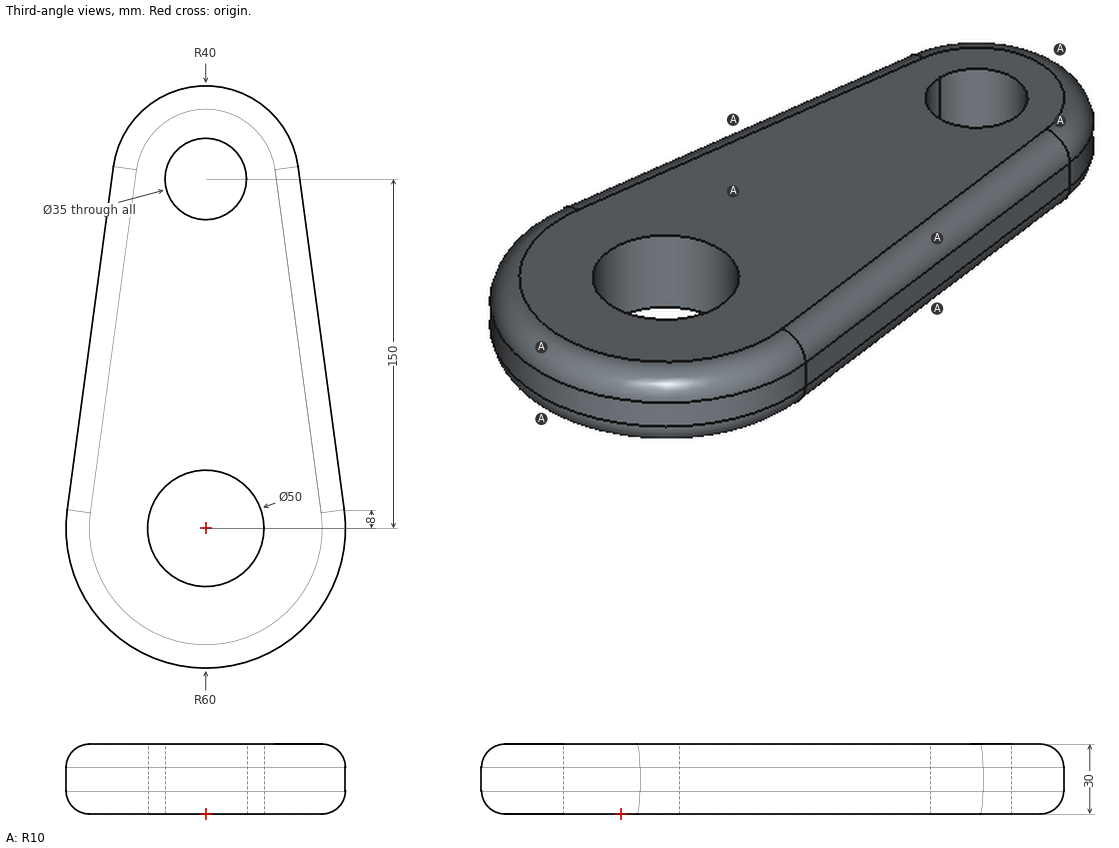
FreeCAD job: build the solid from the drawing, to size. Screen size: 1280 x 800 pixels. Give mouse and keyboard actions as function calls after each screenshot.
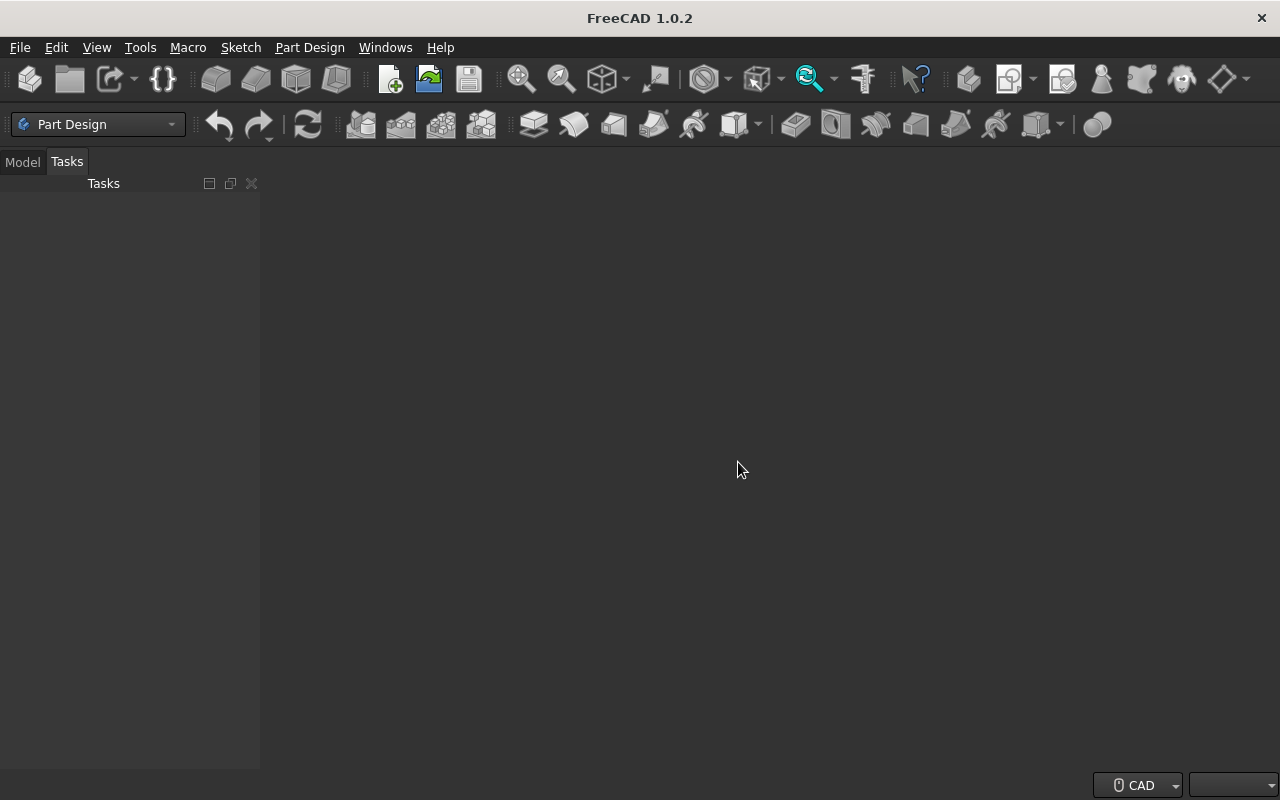
click(390, 80)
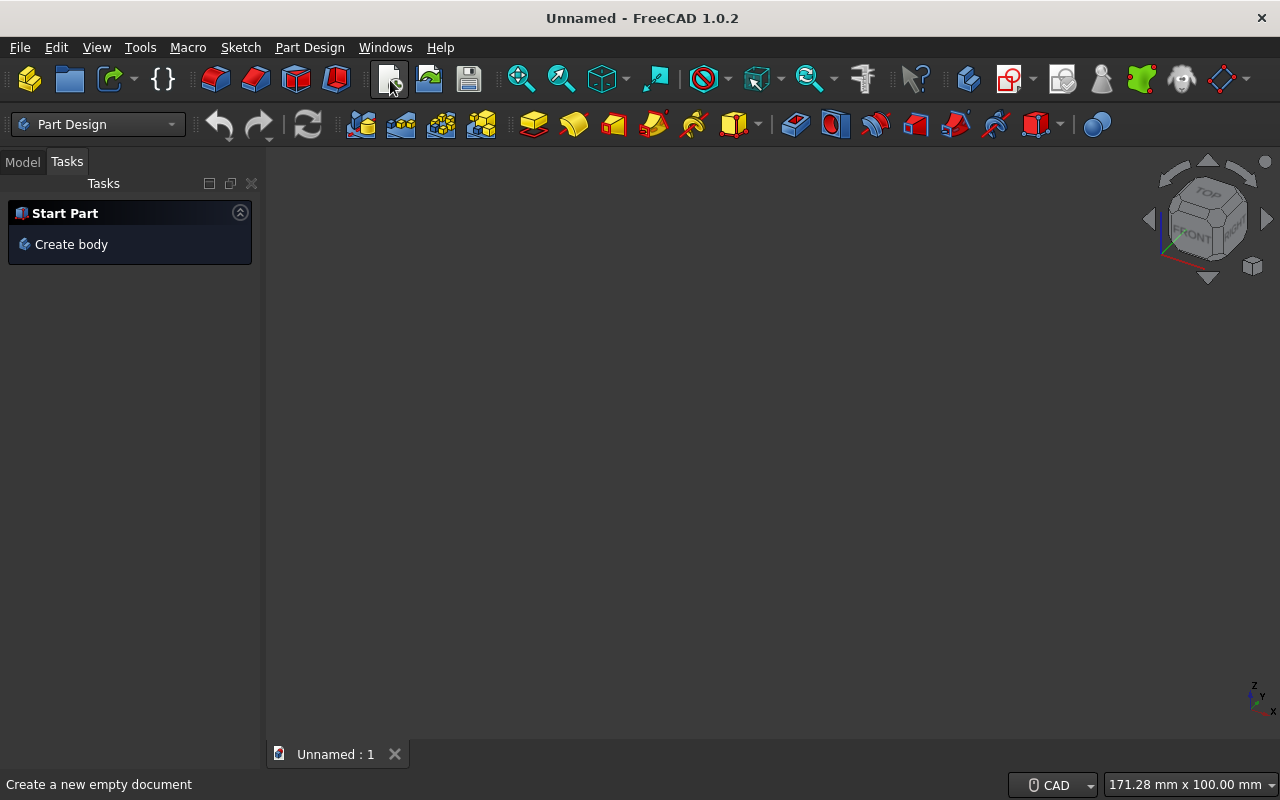
click(970, 80)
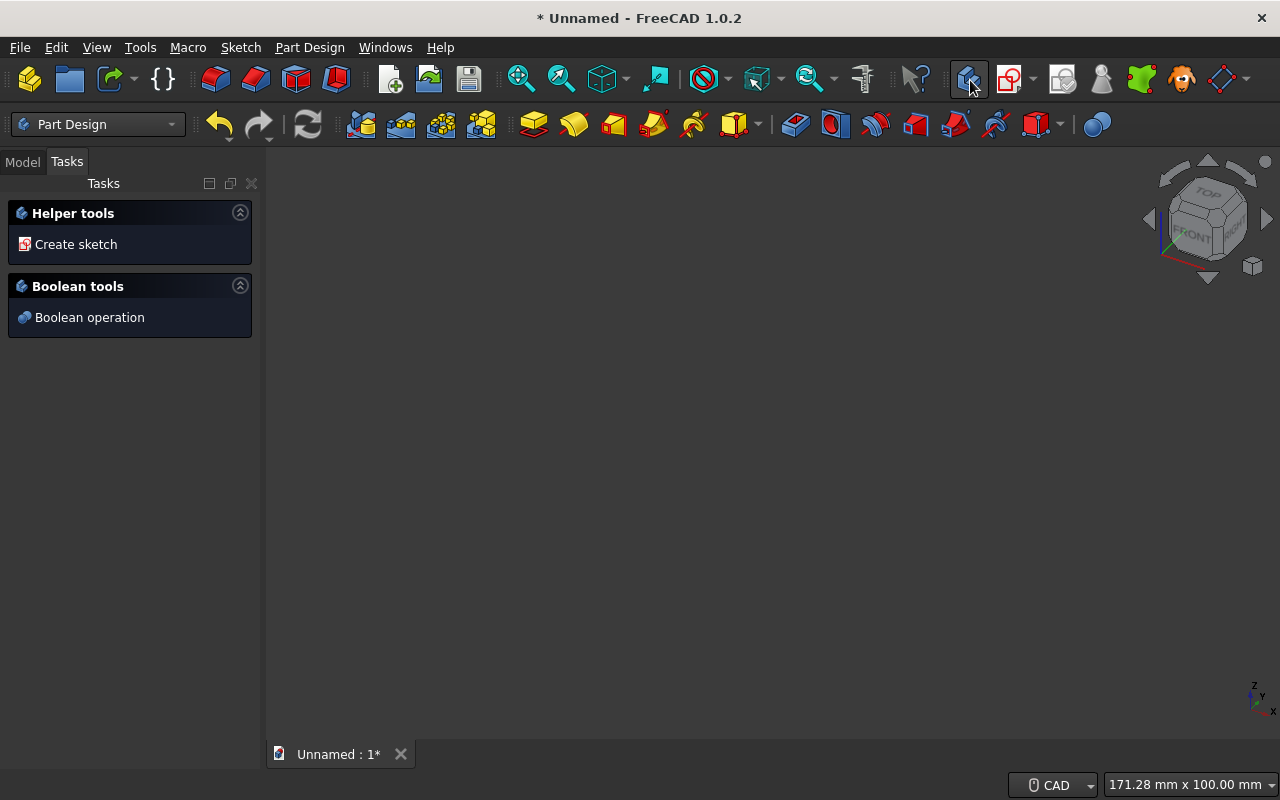
click(23, 161)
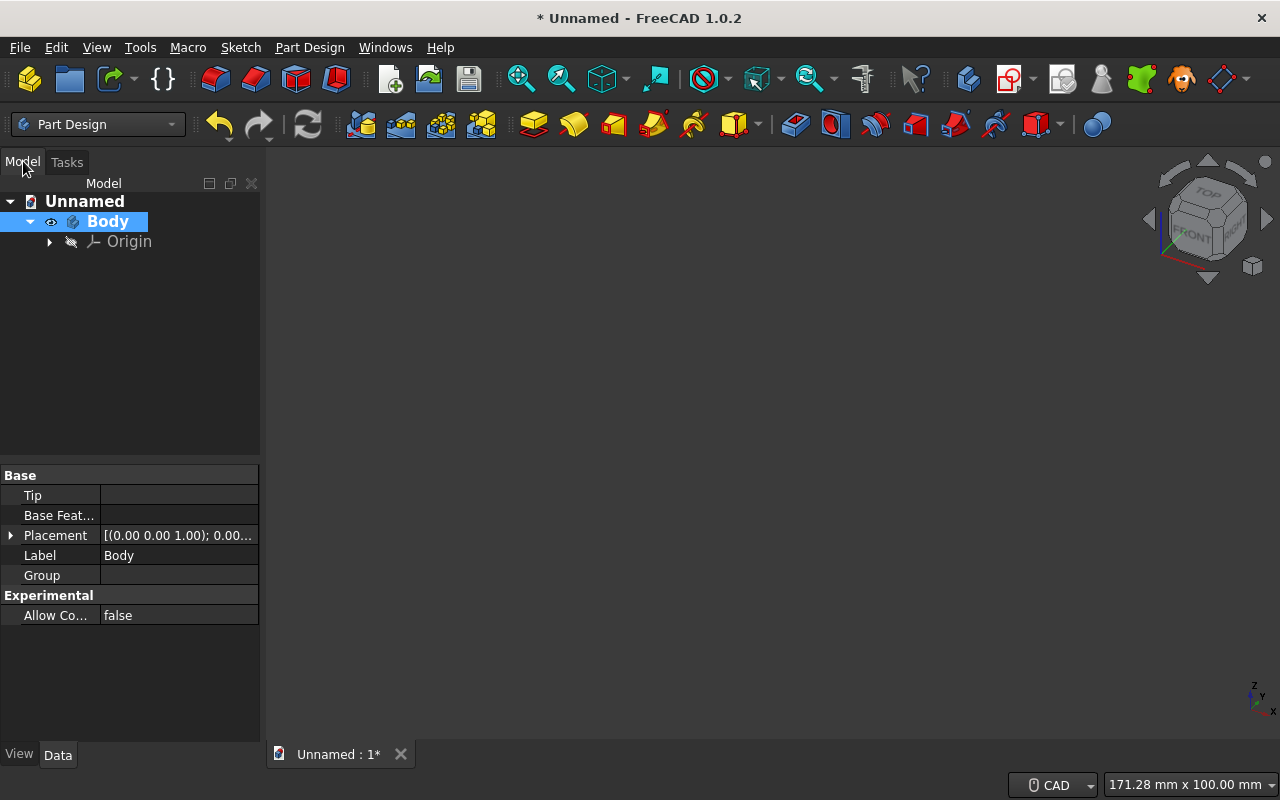
click(50, 242)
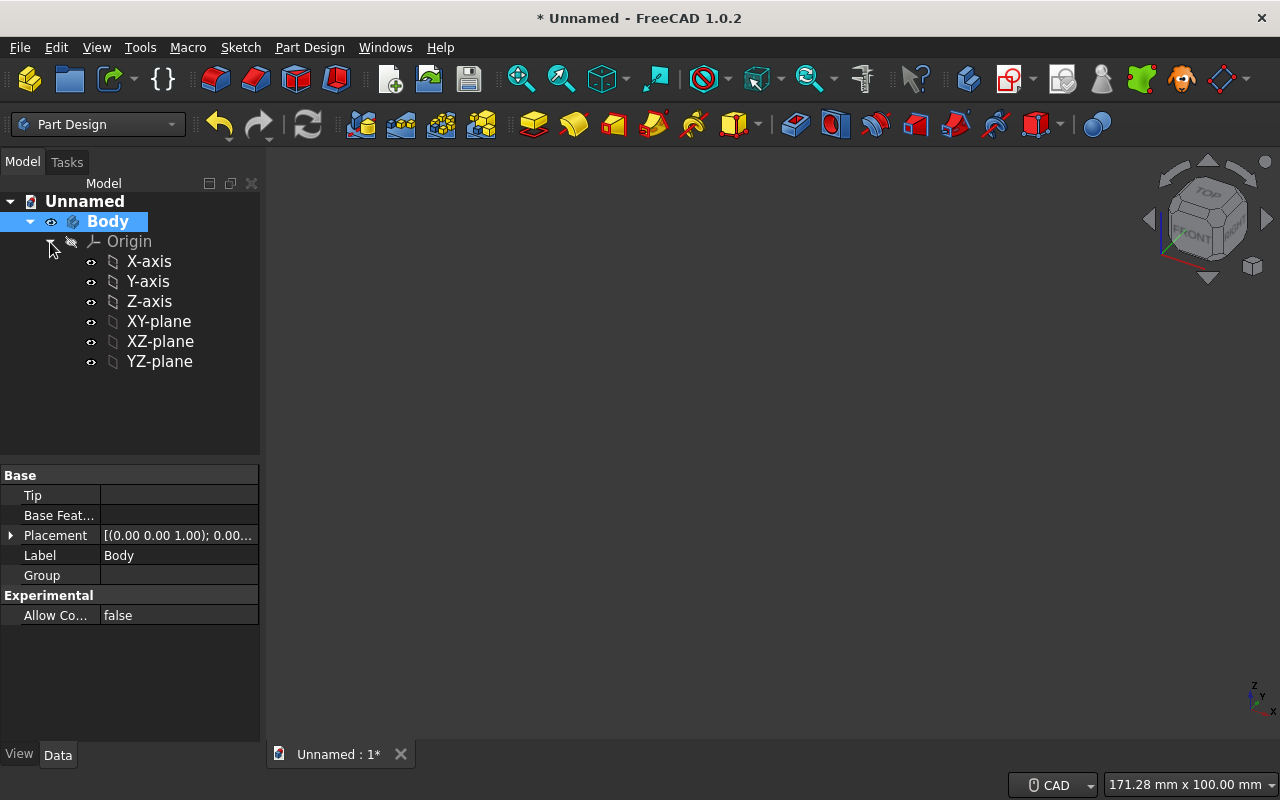
click(136, 322)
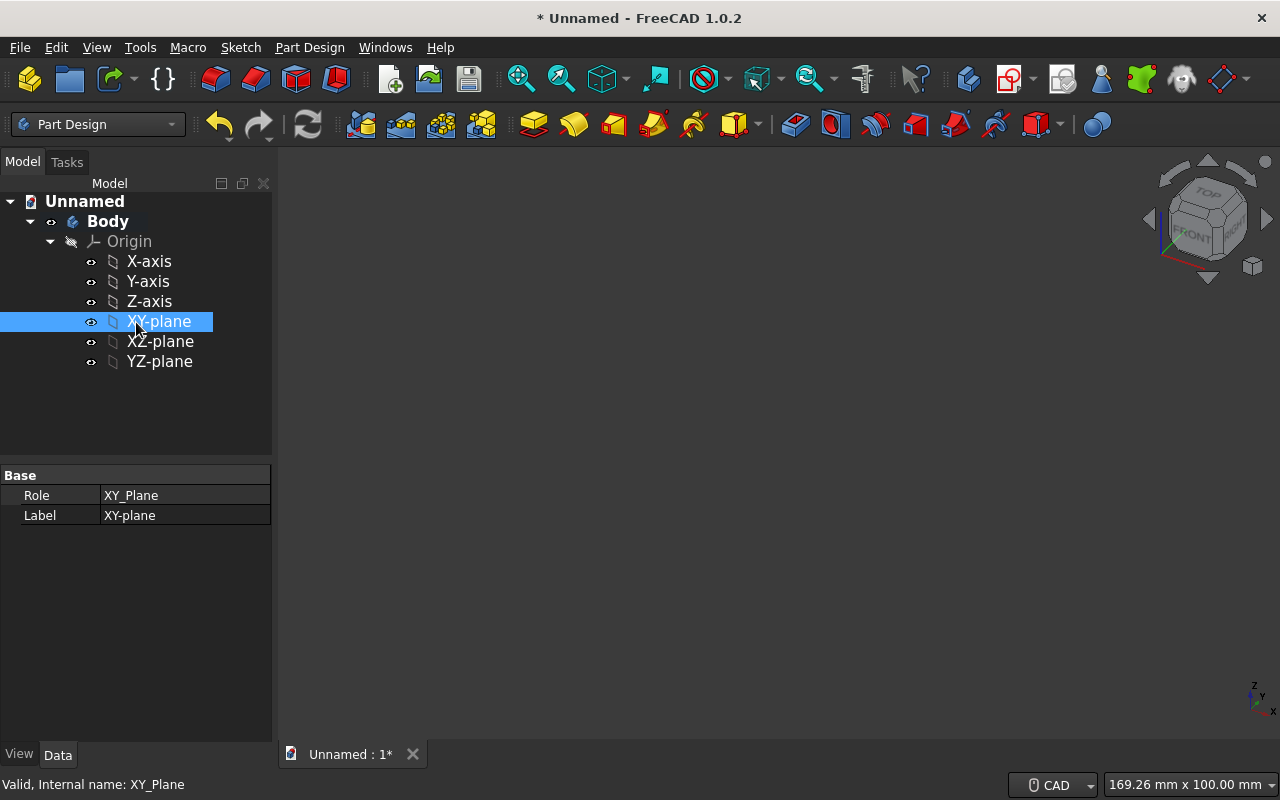
click(1222, 80)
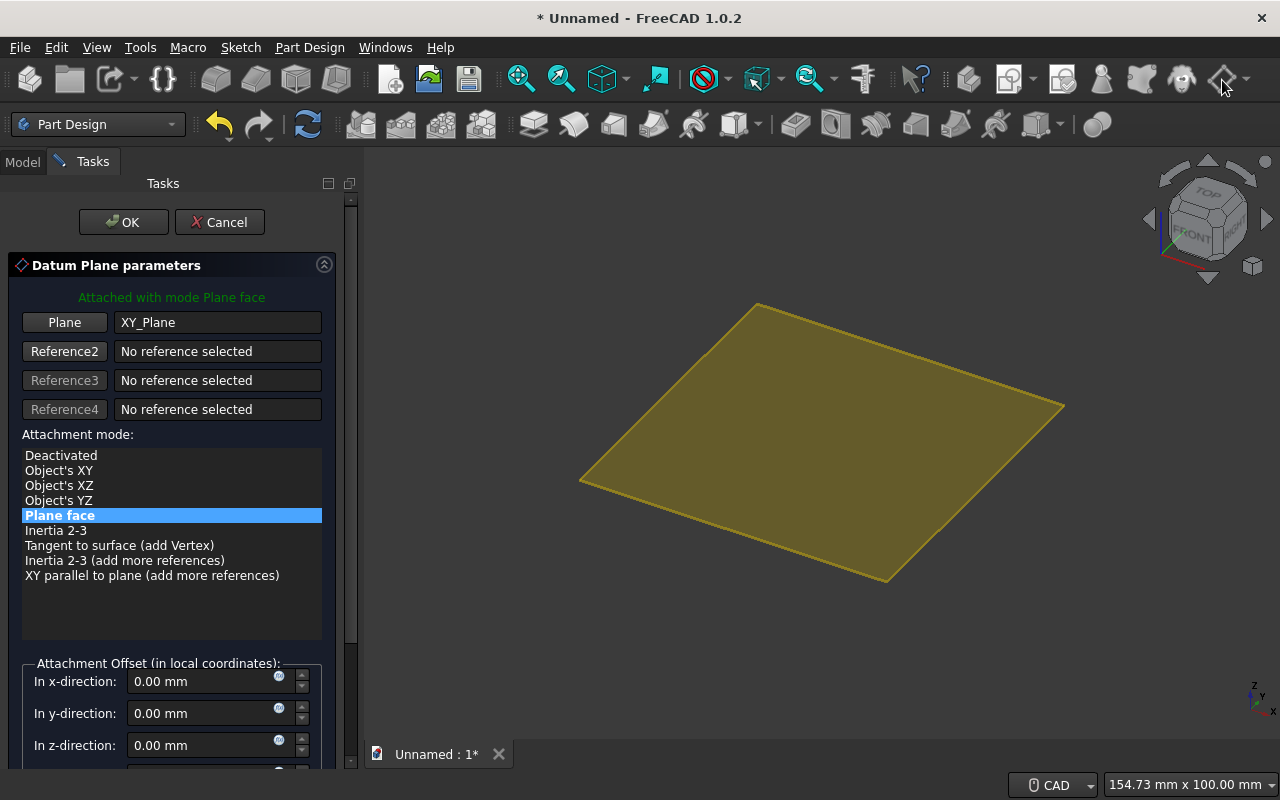
triple_click(210, 745)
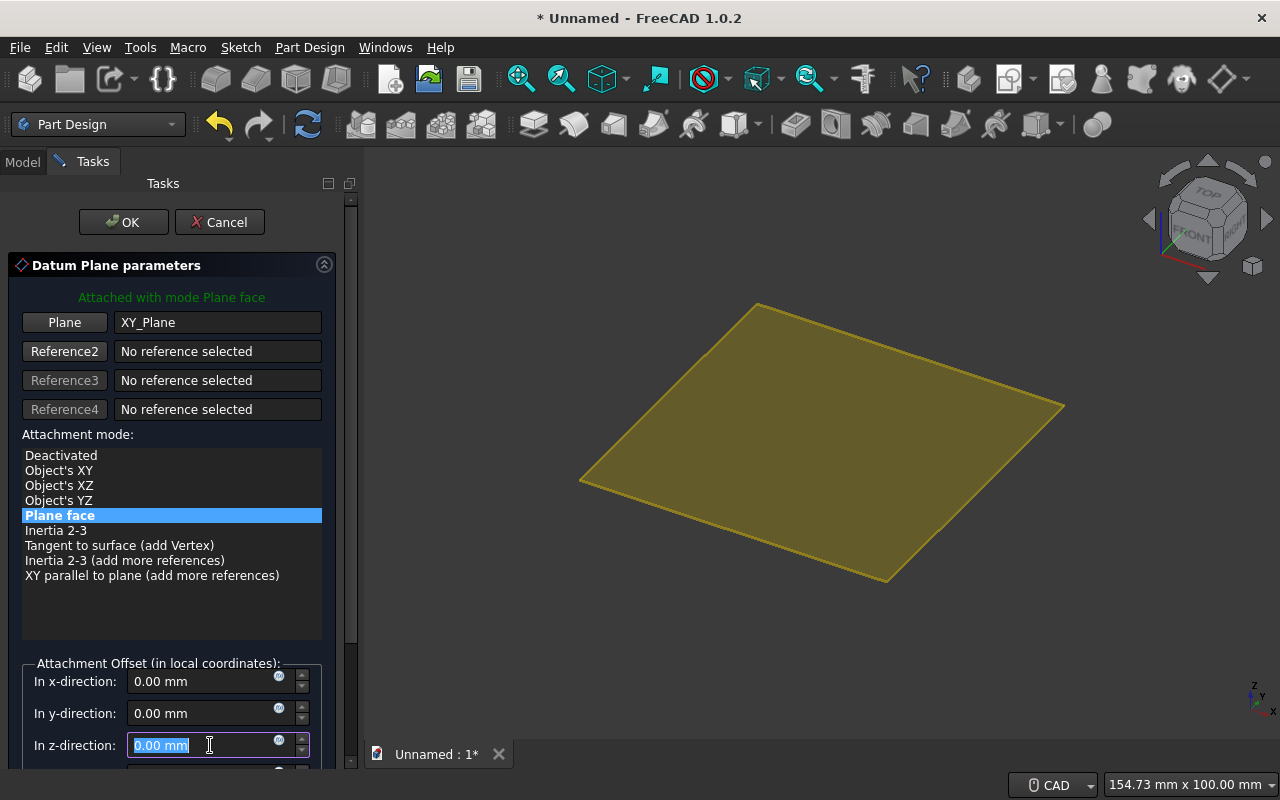
text(30)
key(Tab)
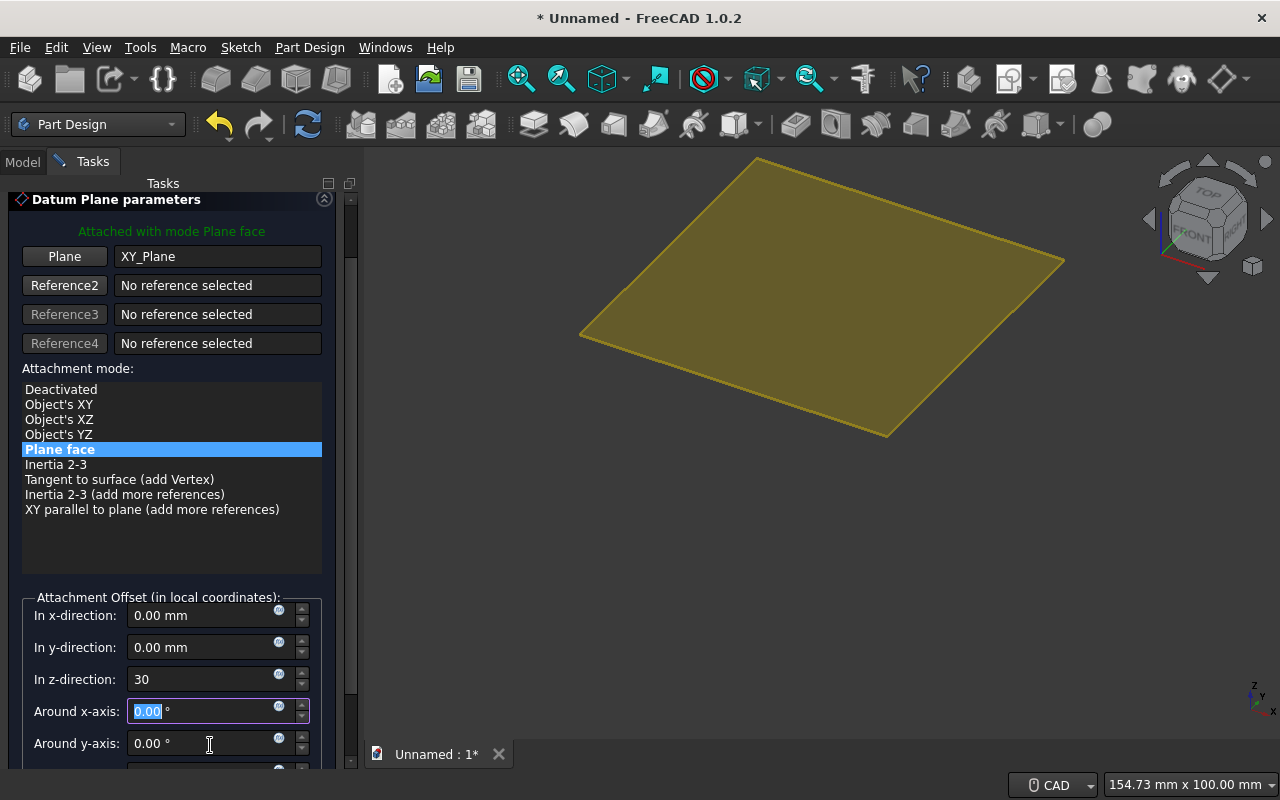
scroll(351, 480, up, 2)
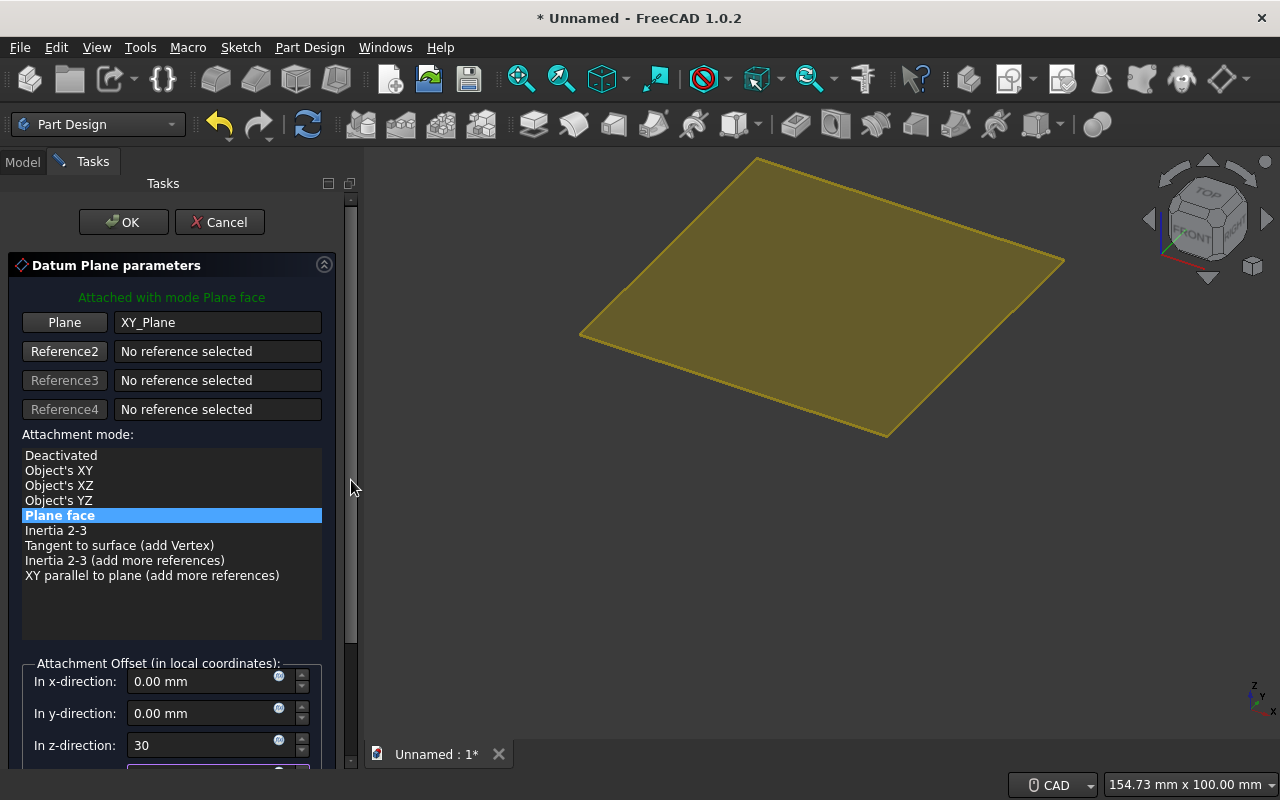
click(124, 222)